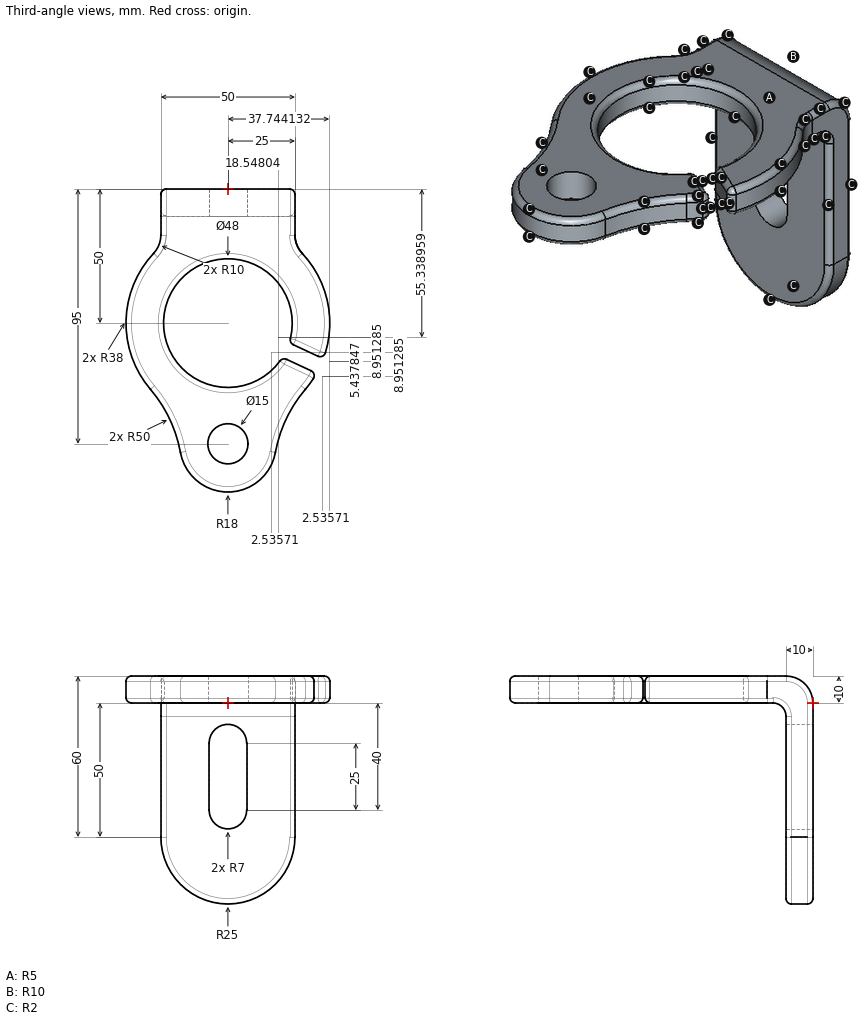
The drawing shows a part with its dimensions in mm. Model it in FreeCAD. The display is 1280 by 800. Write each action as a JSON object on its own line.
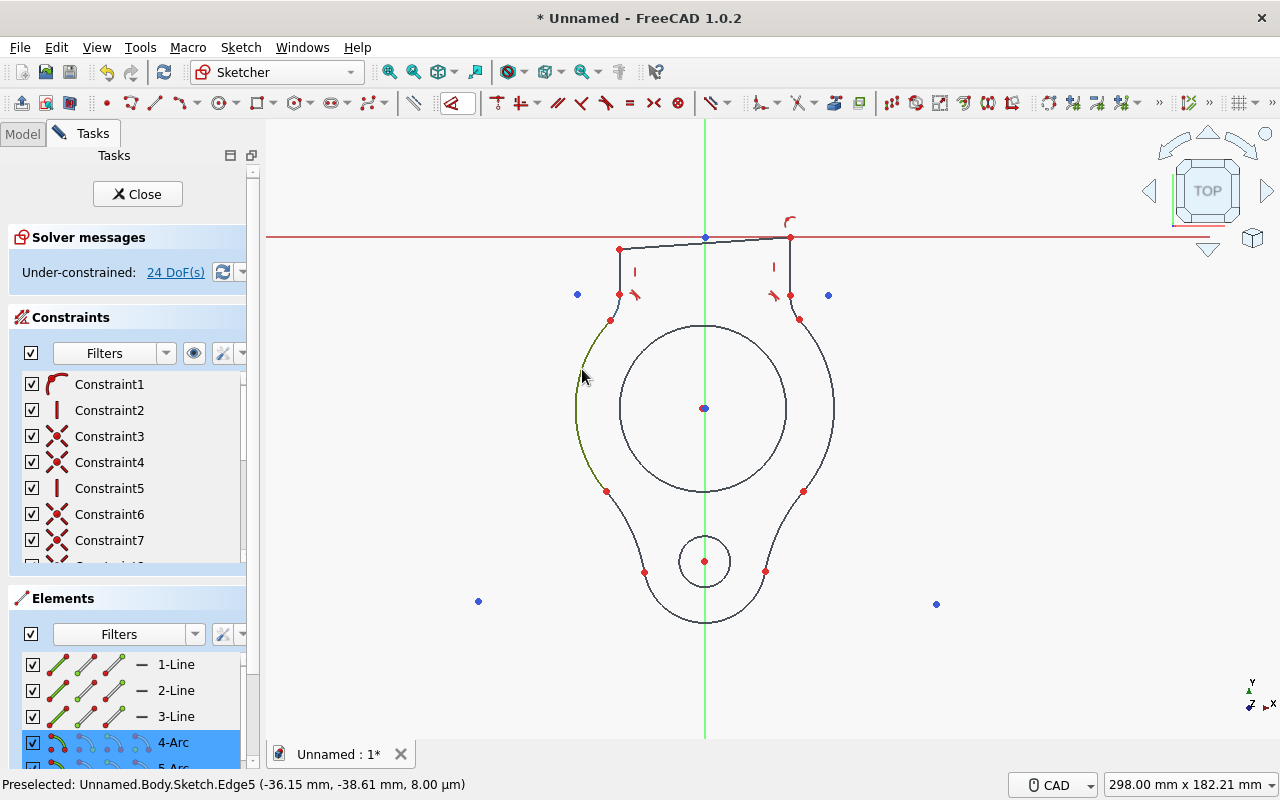
{"action": "left_click", "coordinate": [606, 104]}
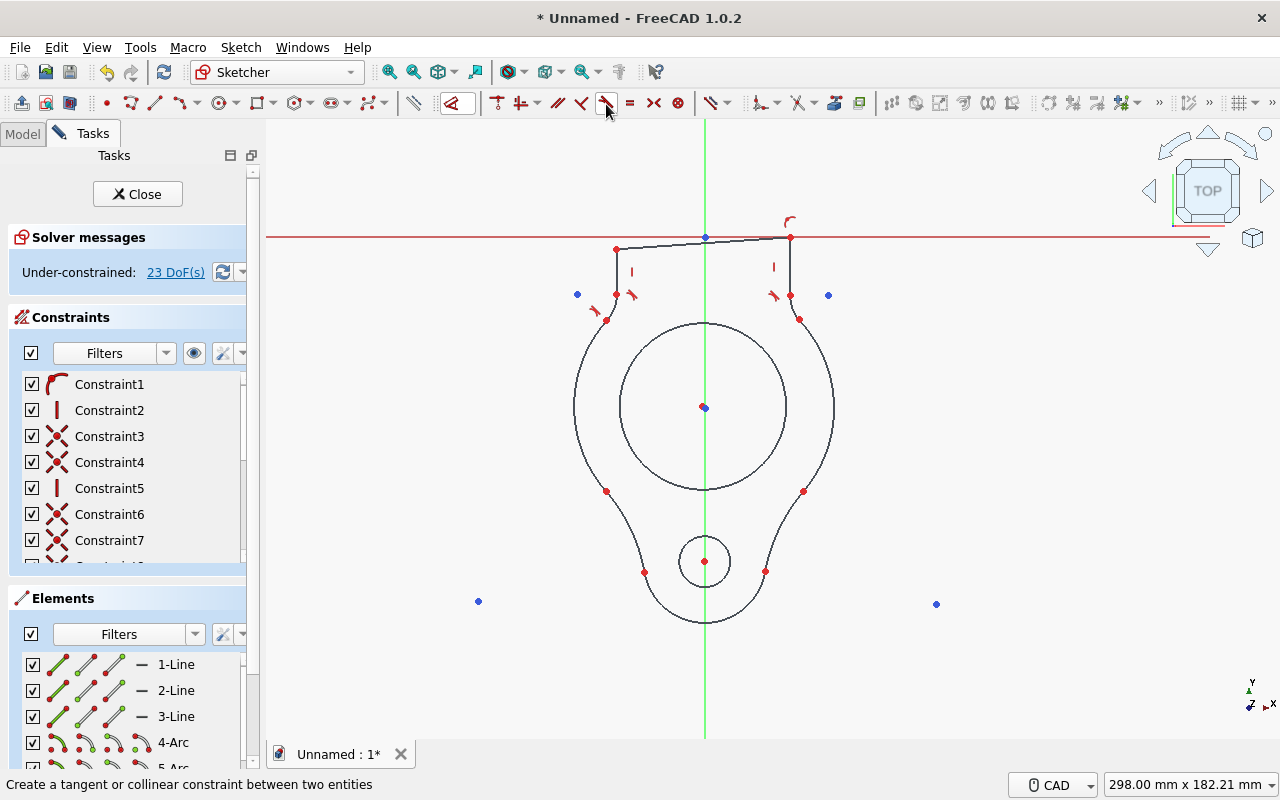
{"action": "left_click", "coordinate": [580, 369]}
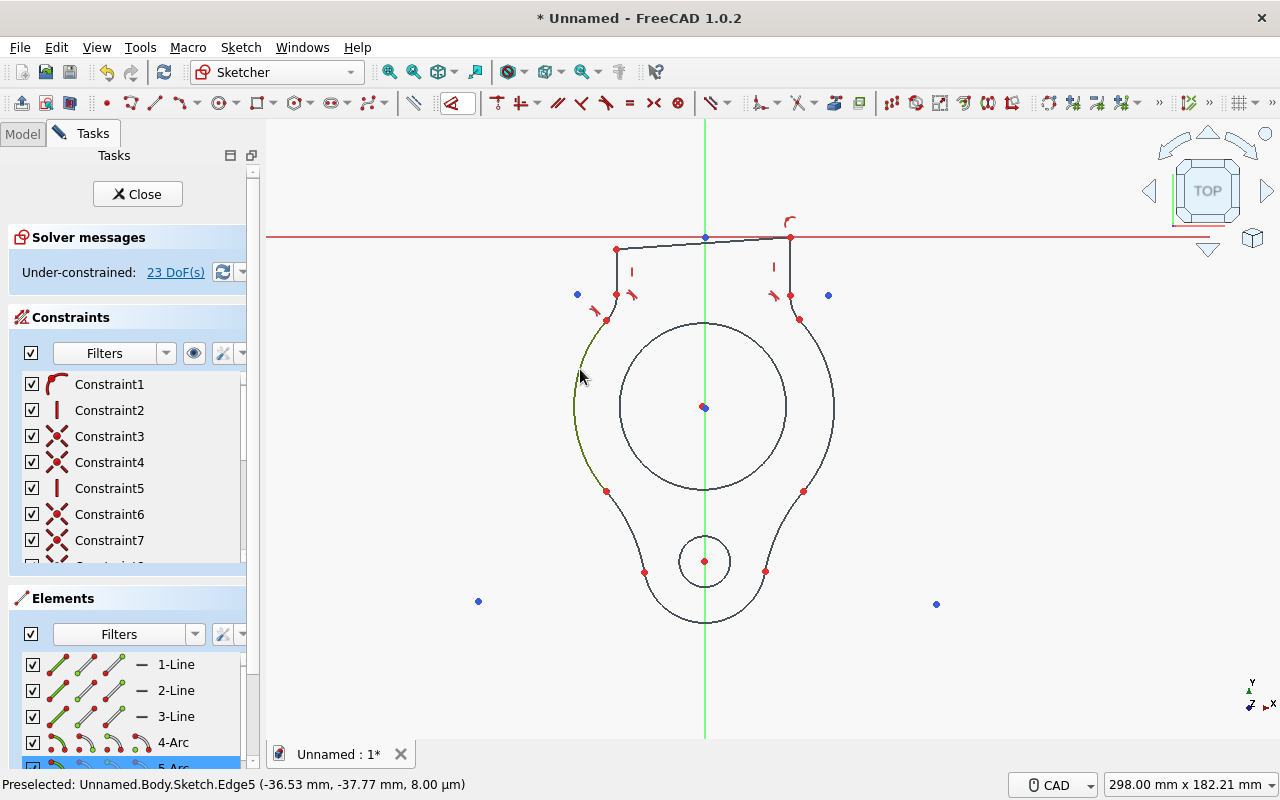
{"action": "left_click", "coordinate": [638, 547]}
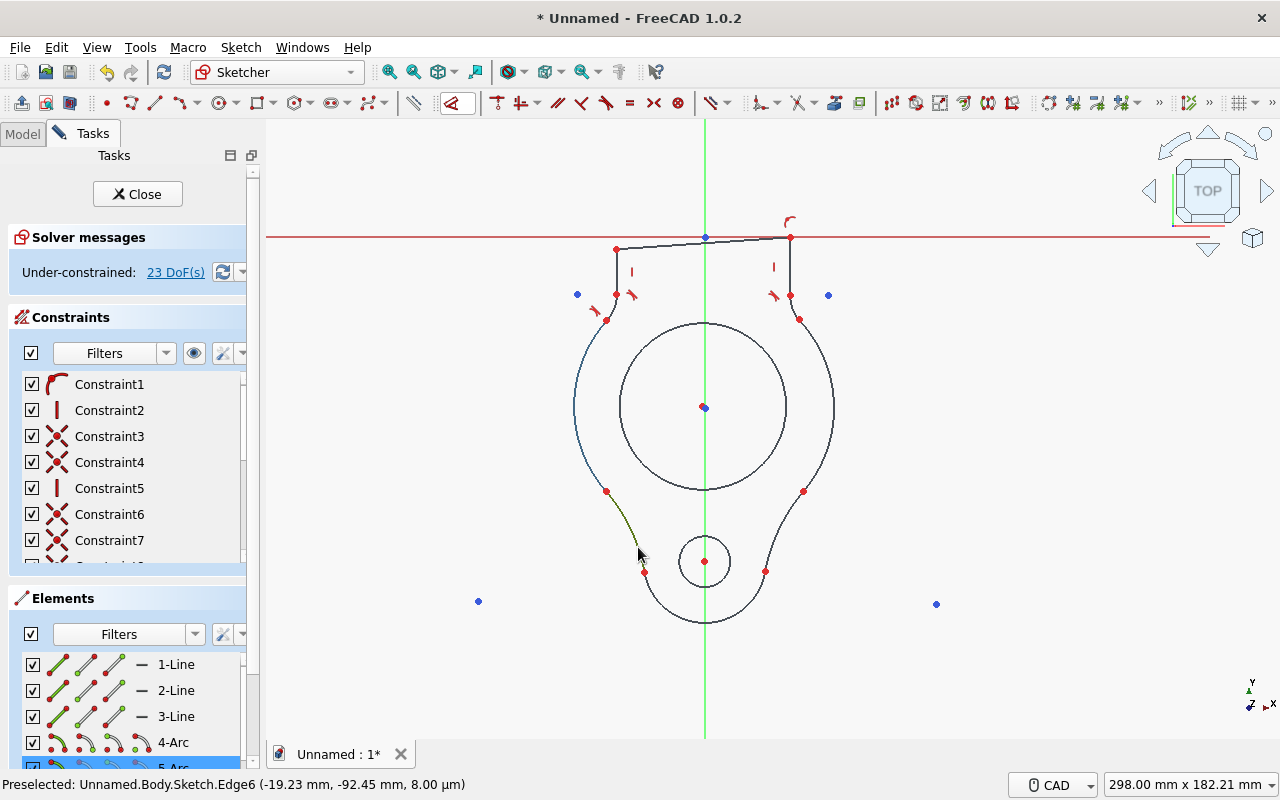
{"action": "left_click", "coordinate": [606, 104]}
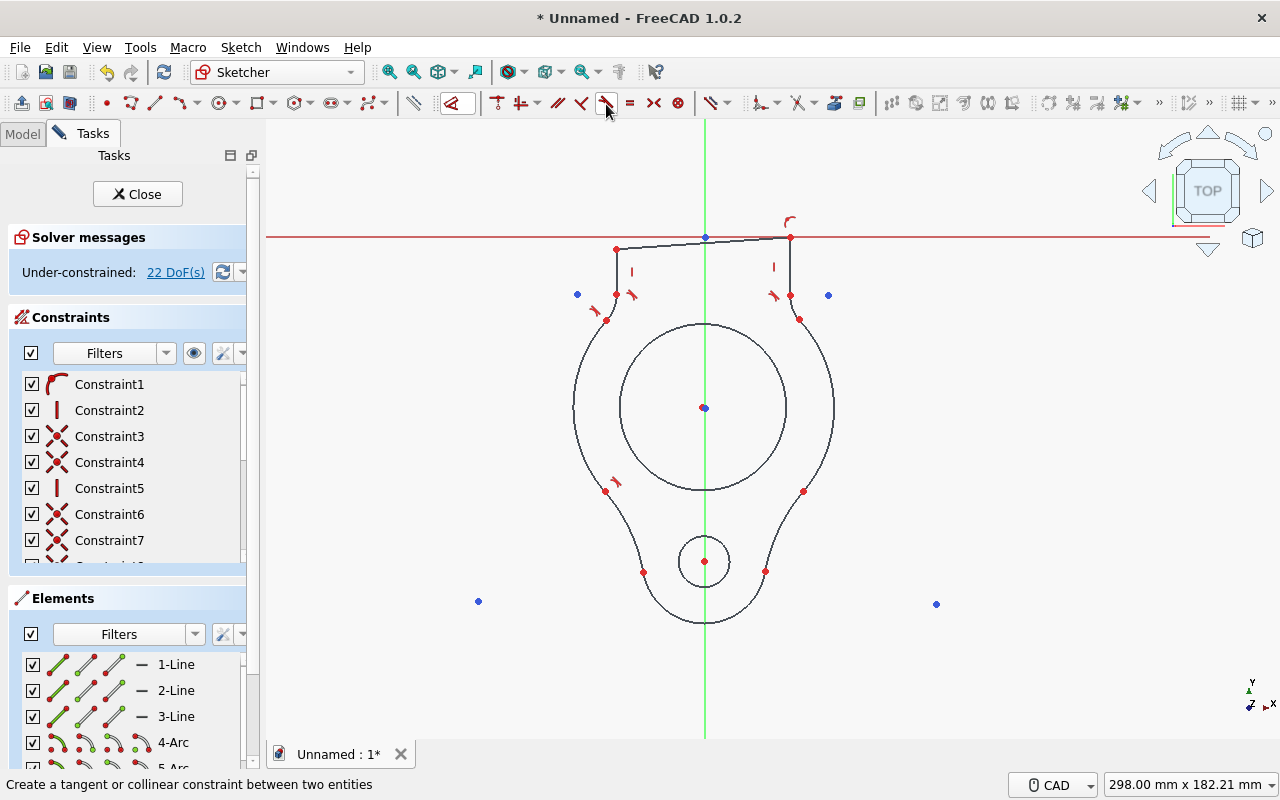
{"action": "left_click", "coordinate": [637, 547]}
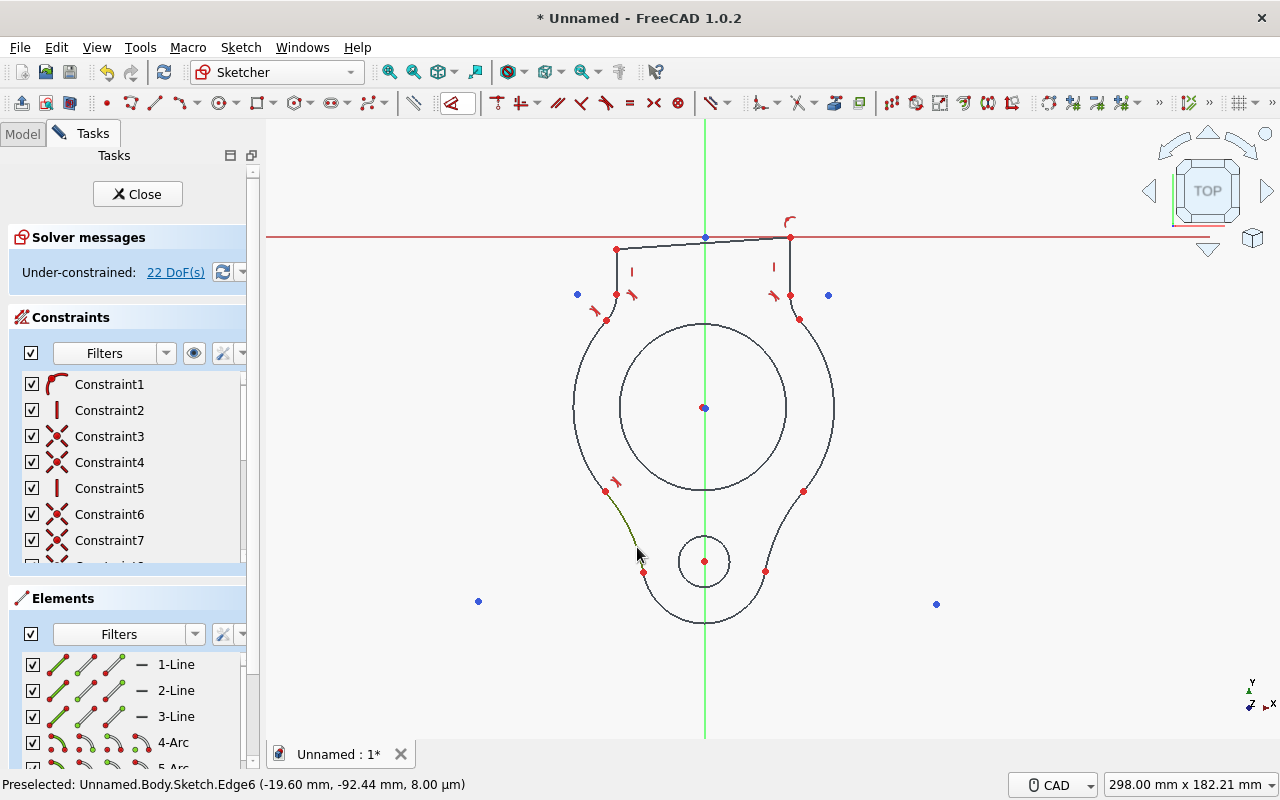
{"action": "left_click", "coordinate": [672, 614]}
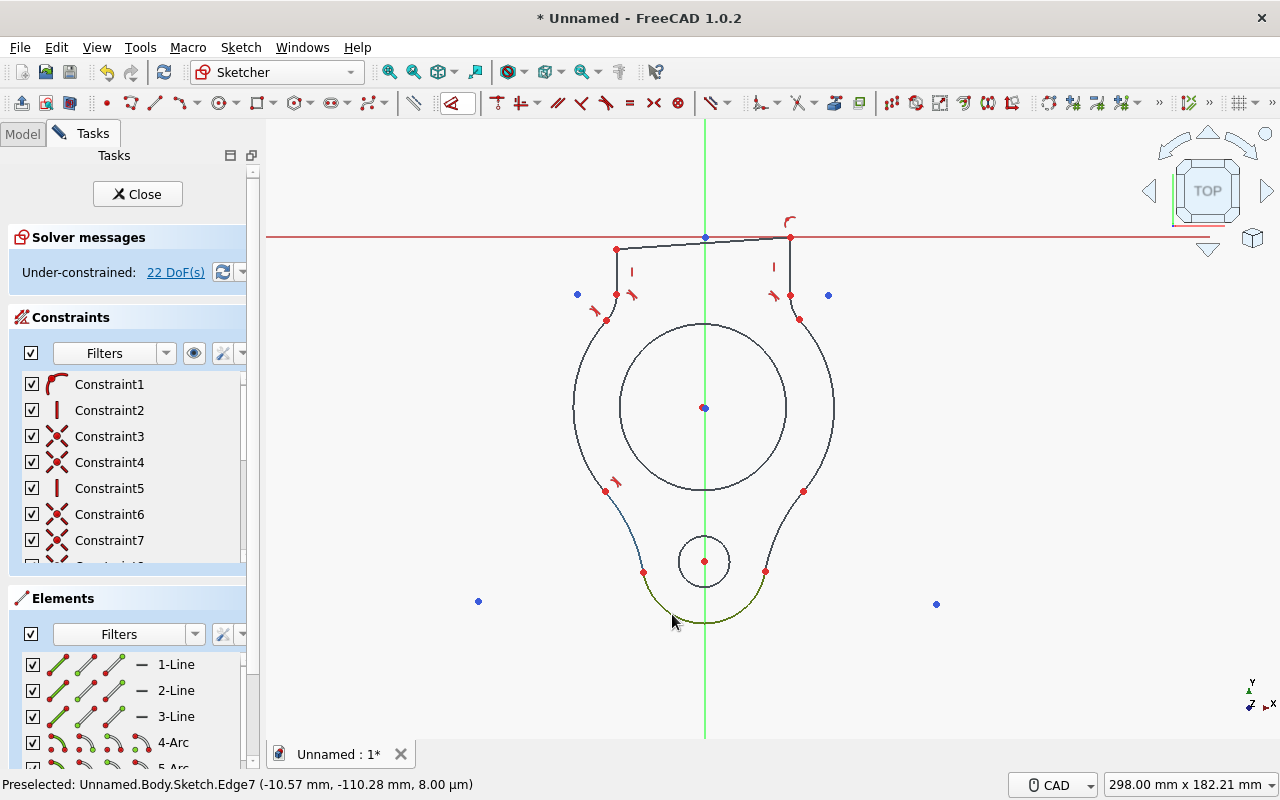
{"action": "left_click", "coordinate": [606, 104]}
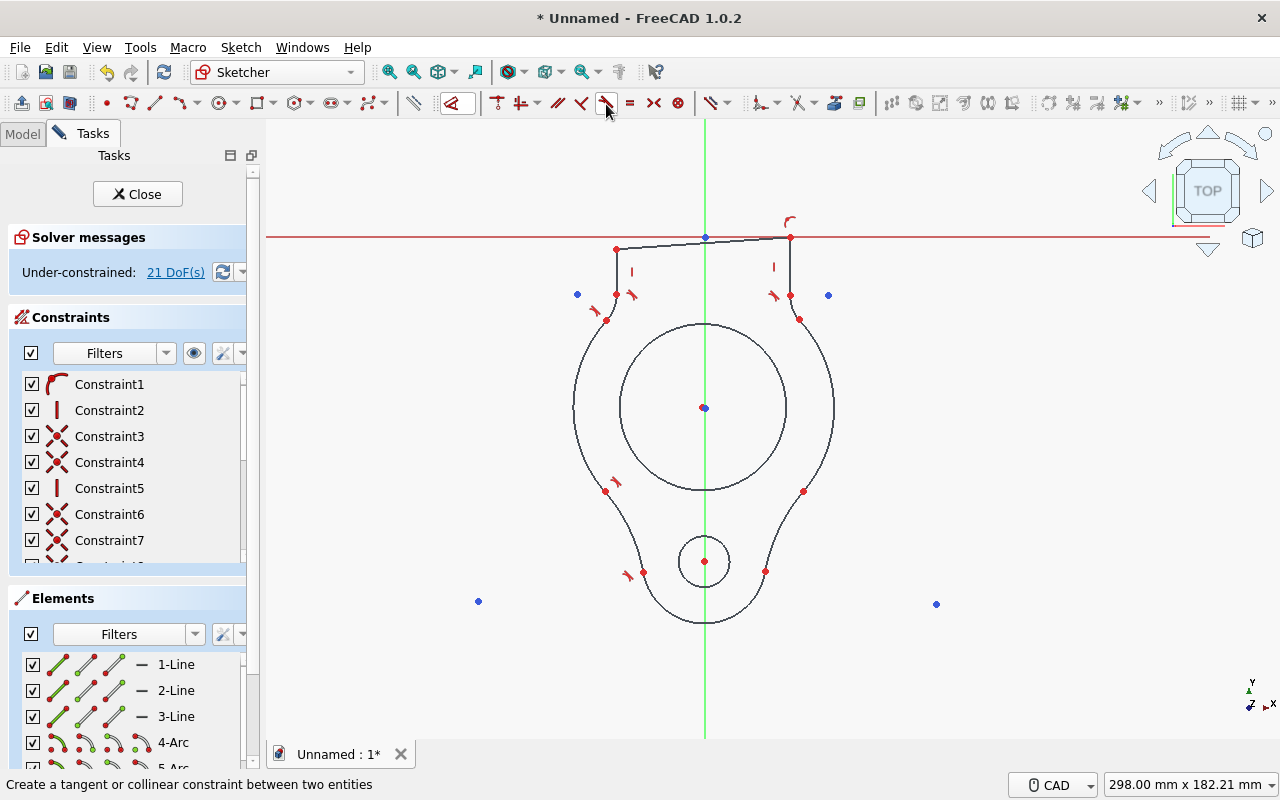
{"action": "left_click", "coordinate": [672, 614]}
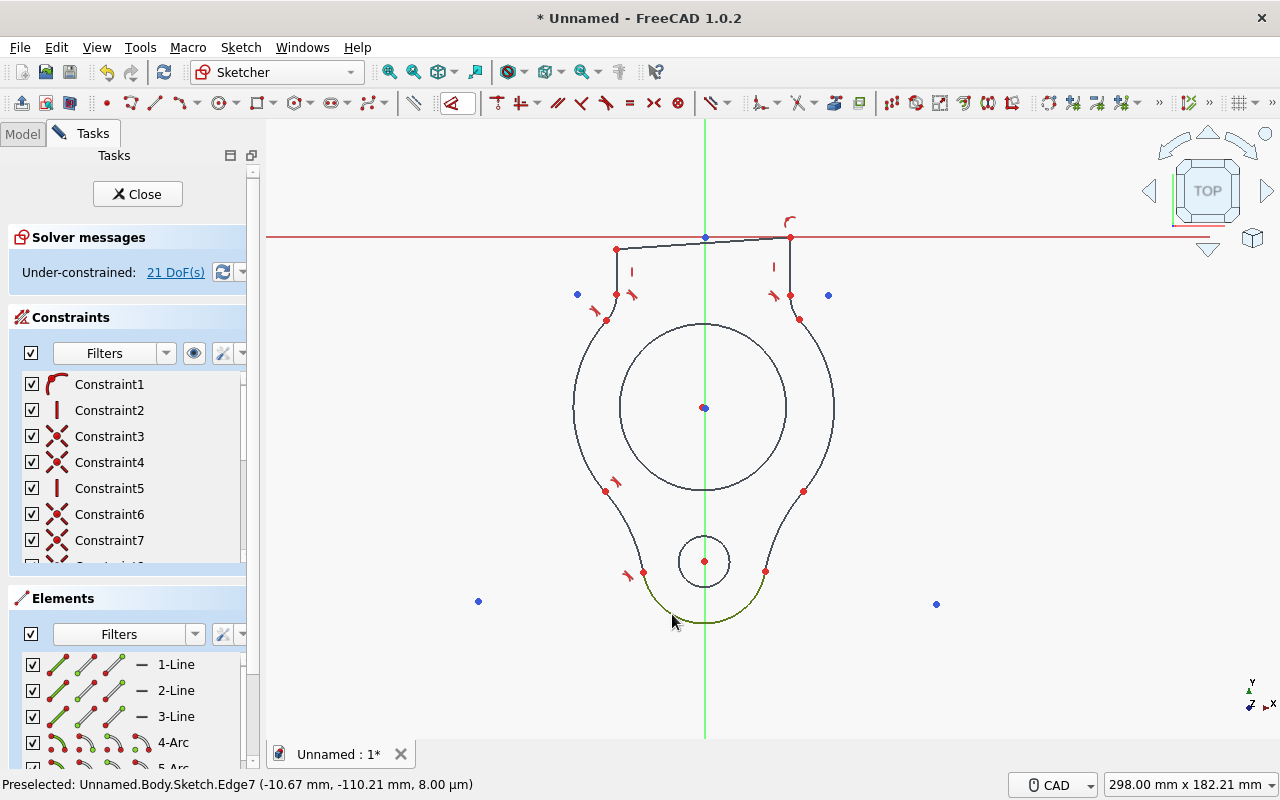
{"action": "left_click", "coordinate": [787, 514]}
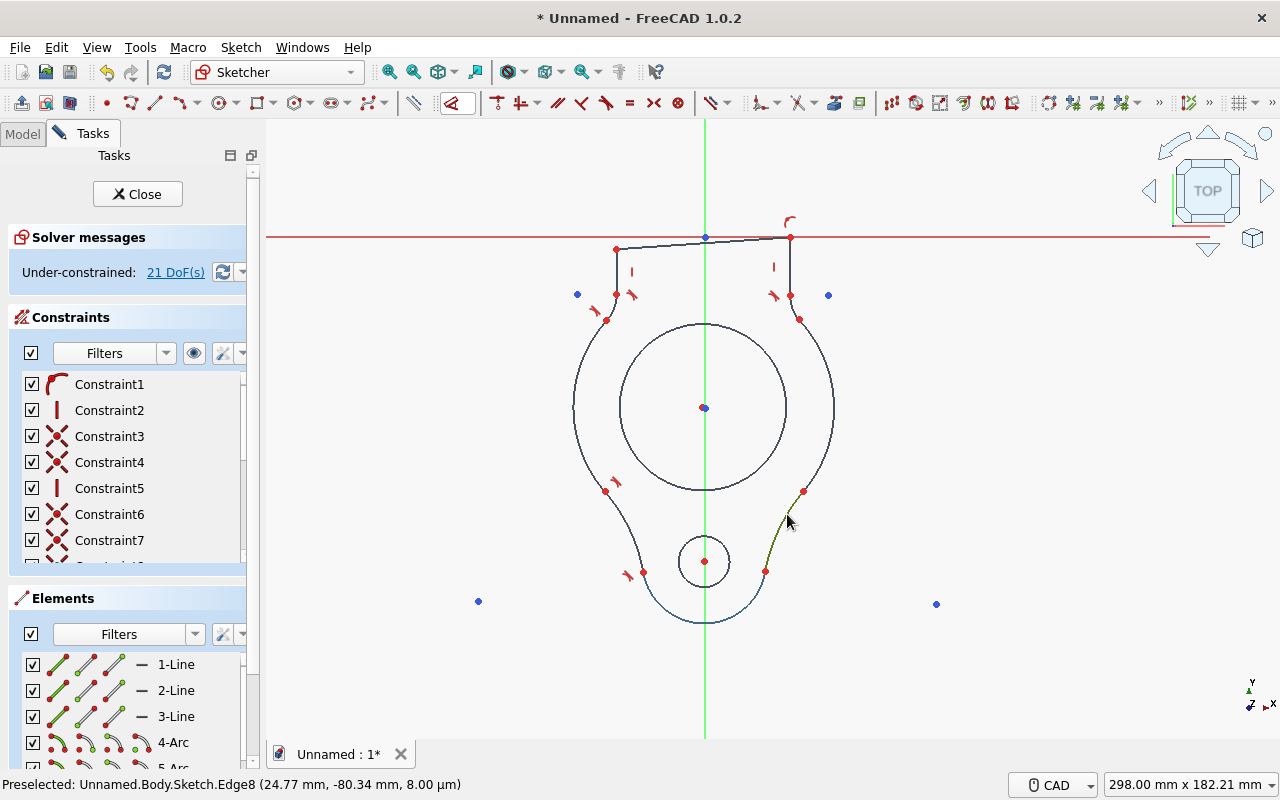
{"action": "left_click", "coordinate": [606, 104]}